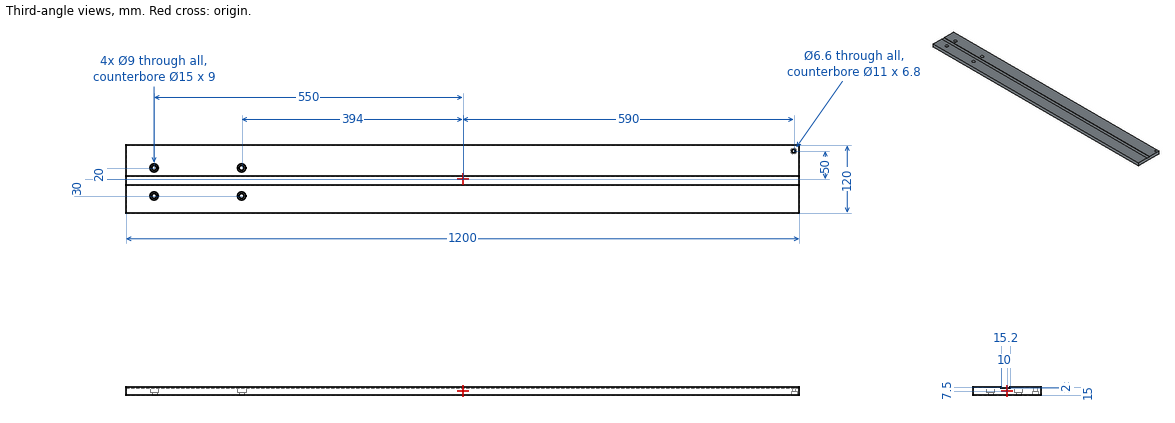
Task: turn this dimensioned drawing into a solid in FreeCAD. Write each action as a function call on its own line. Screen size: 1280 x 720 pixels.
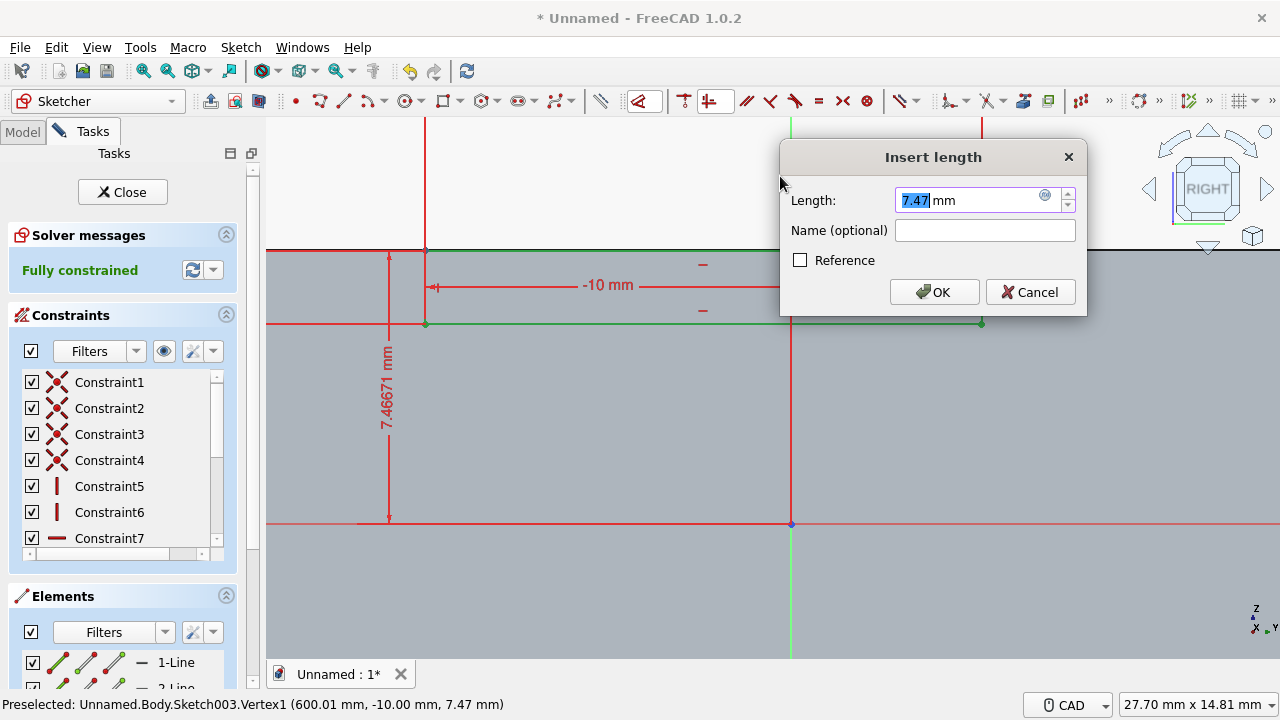
text(7.5)
key(Return)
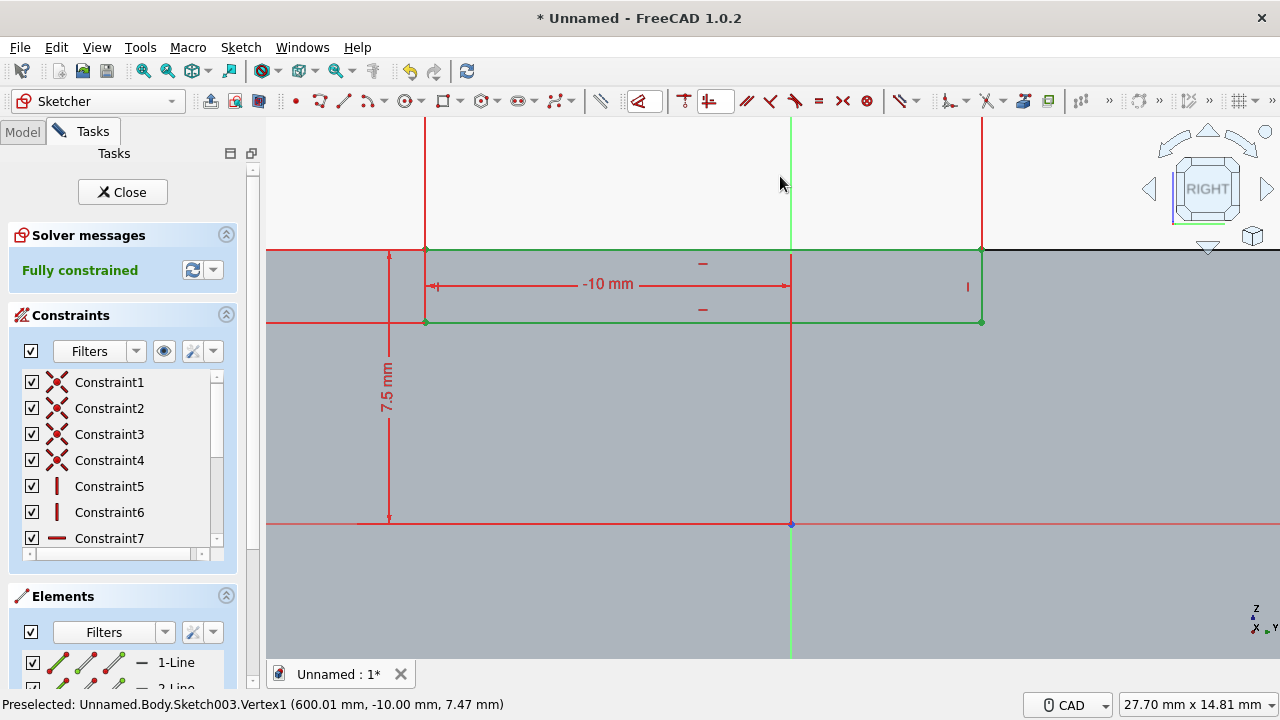
click(123, 192)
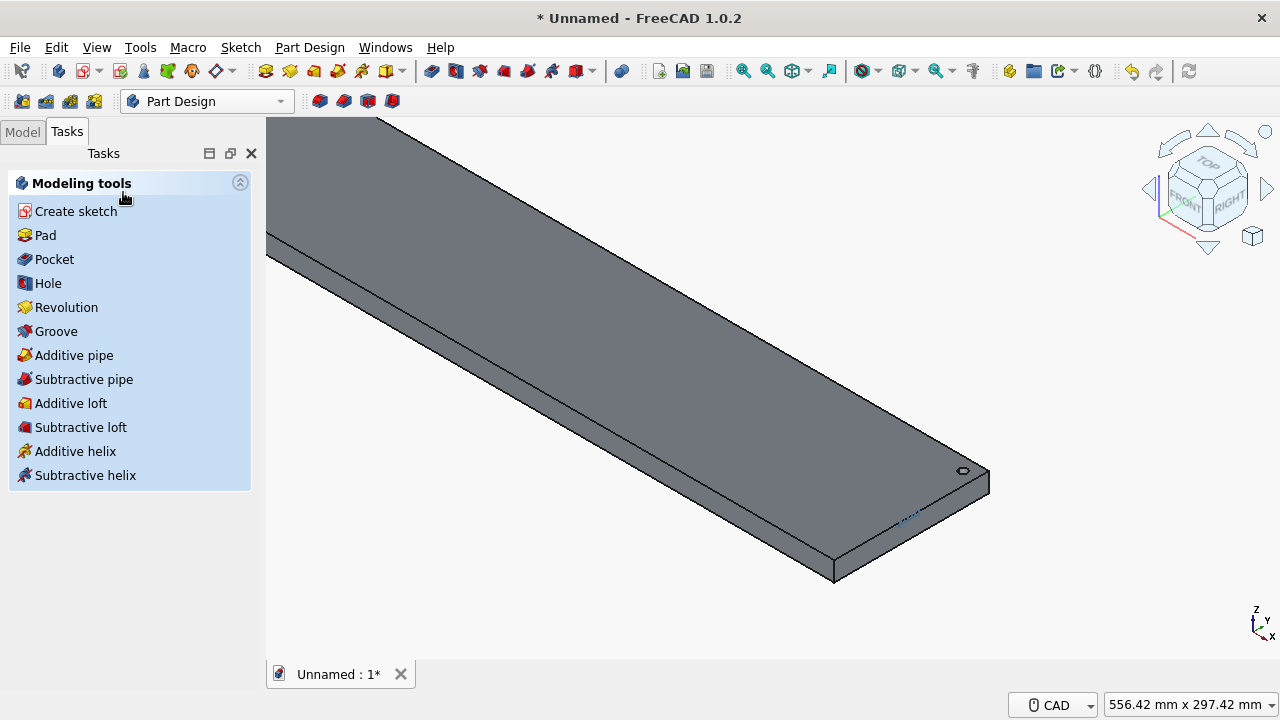
click(432, 72)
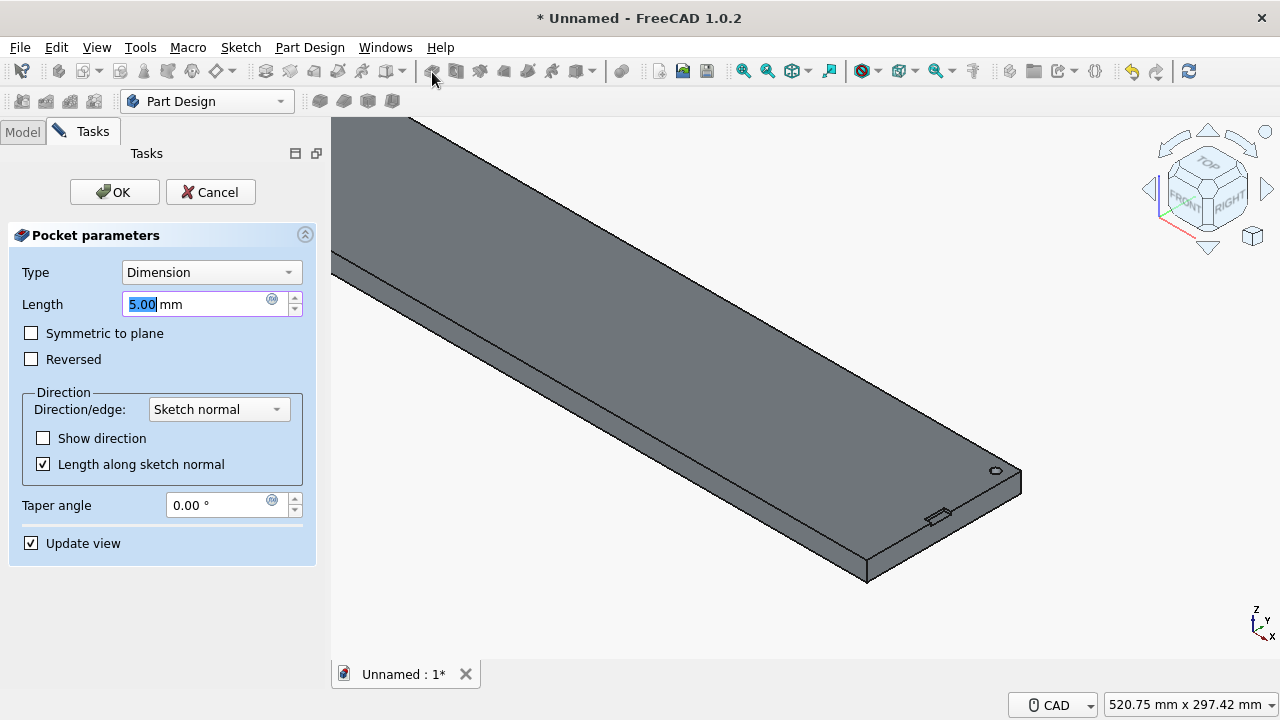
click(212, 272)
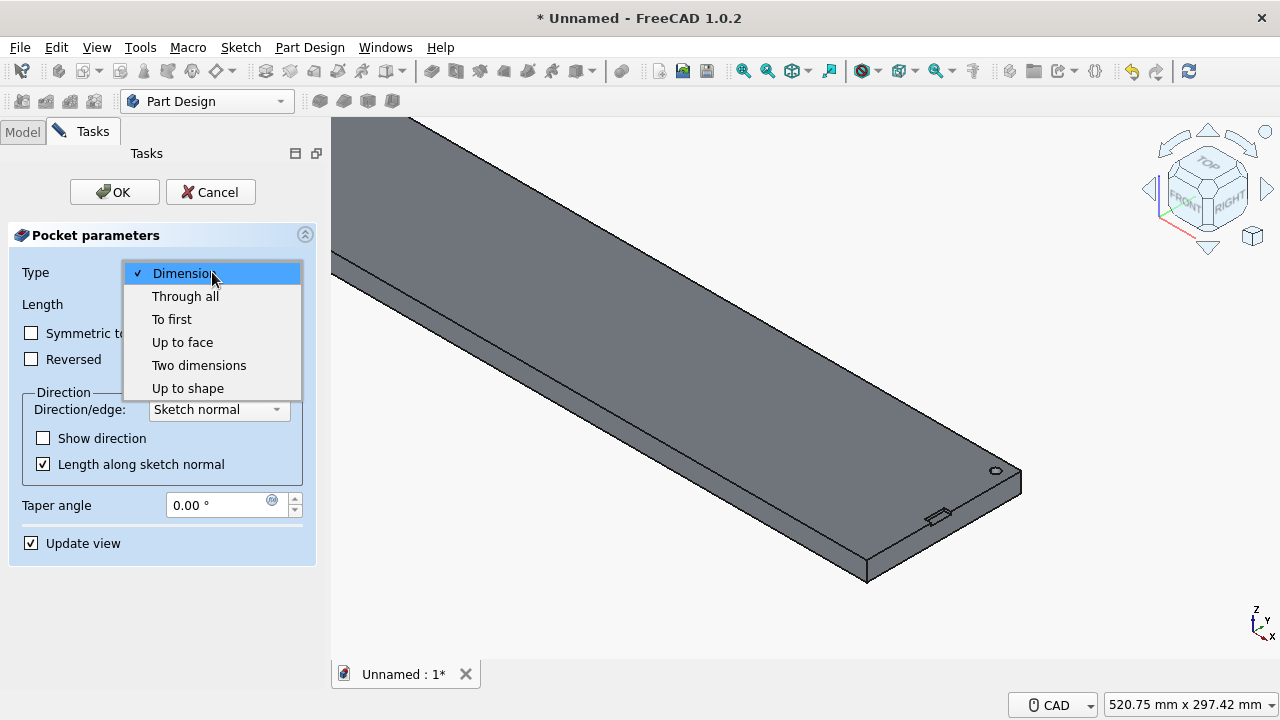
click(212, 296)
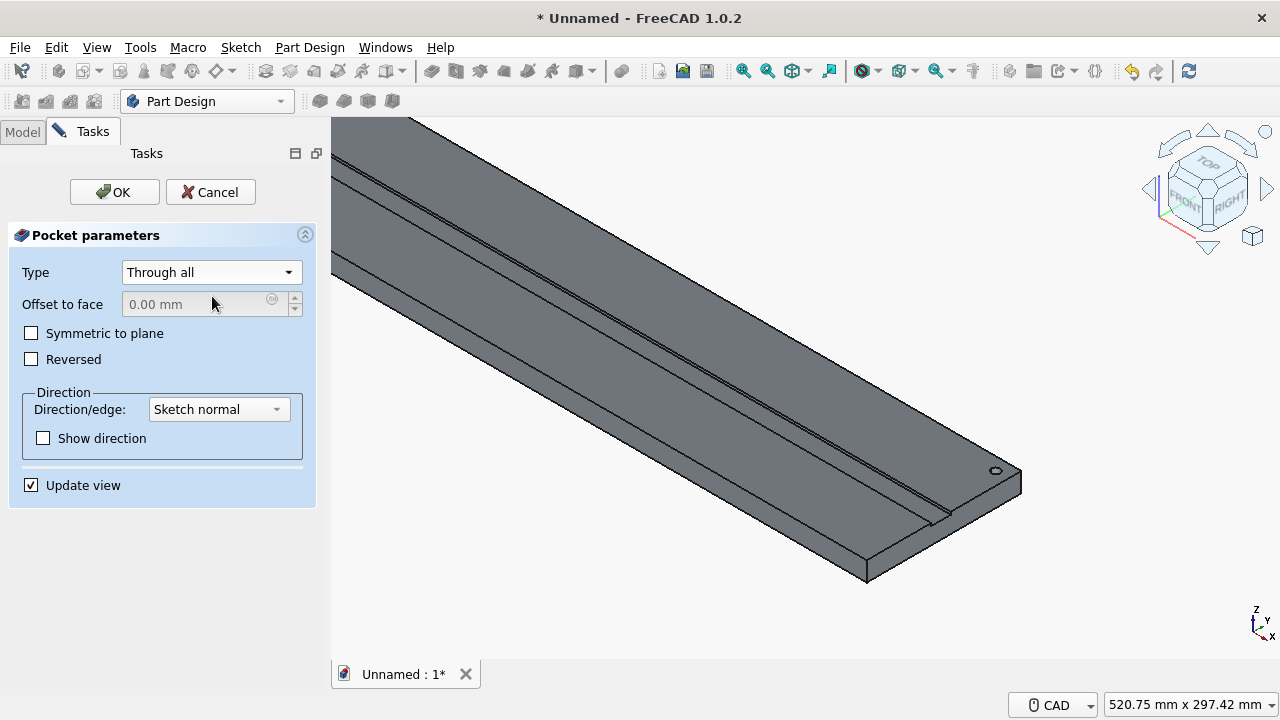
click(115, 192)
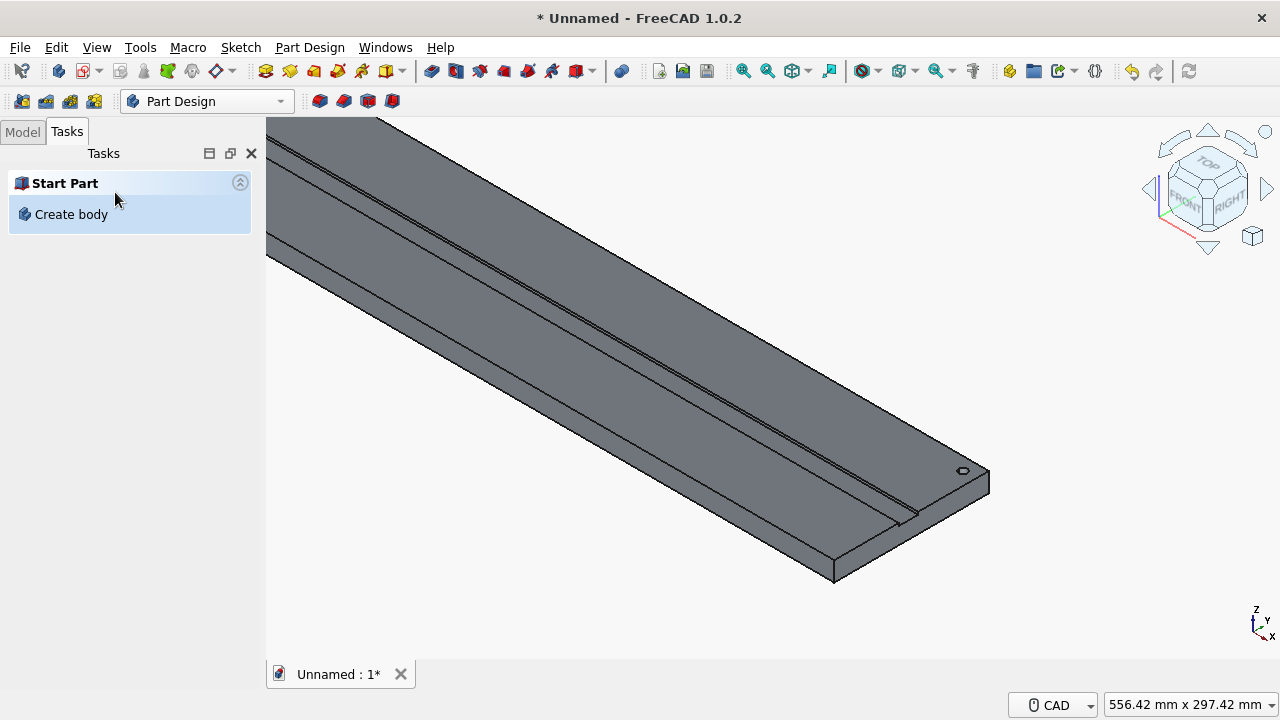
click(744, 72)